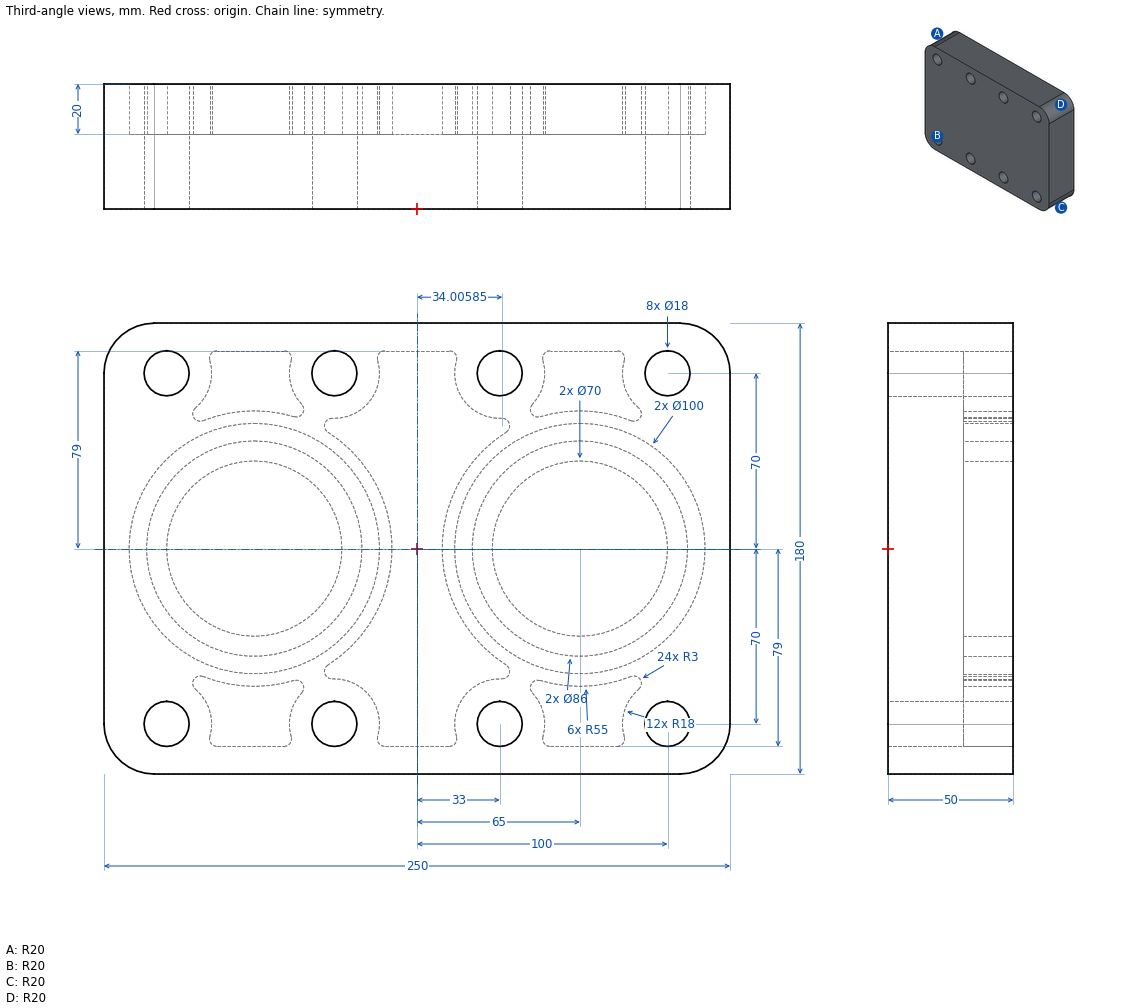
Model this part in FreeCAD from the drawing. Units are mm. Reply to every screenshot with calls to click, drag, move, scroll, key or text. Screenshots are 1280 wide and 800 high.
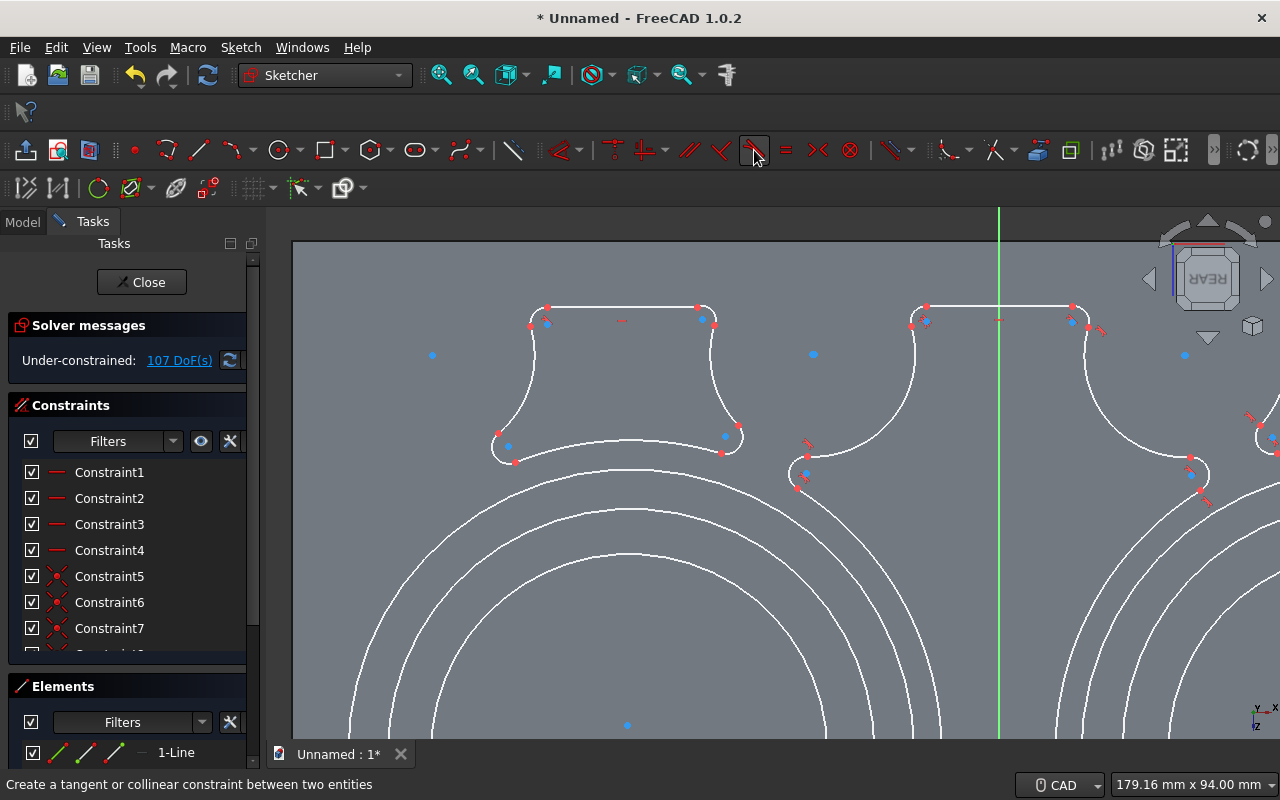
click(652, 307)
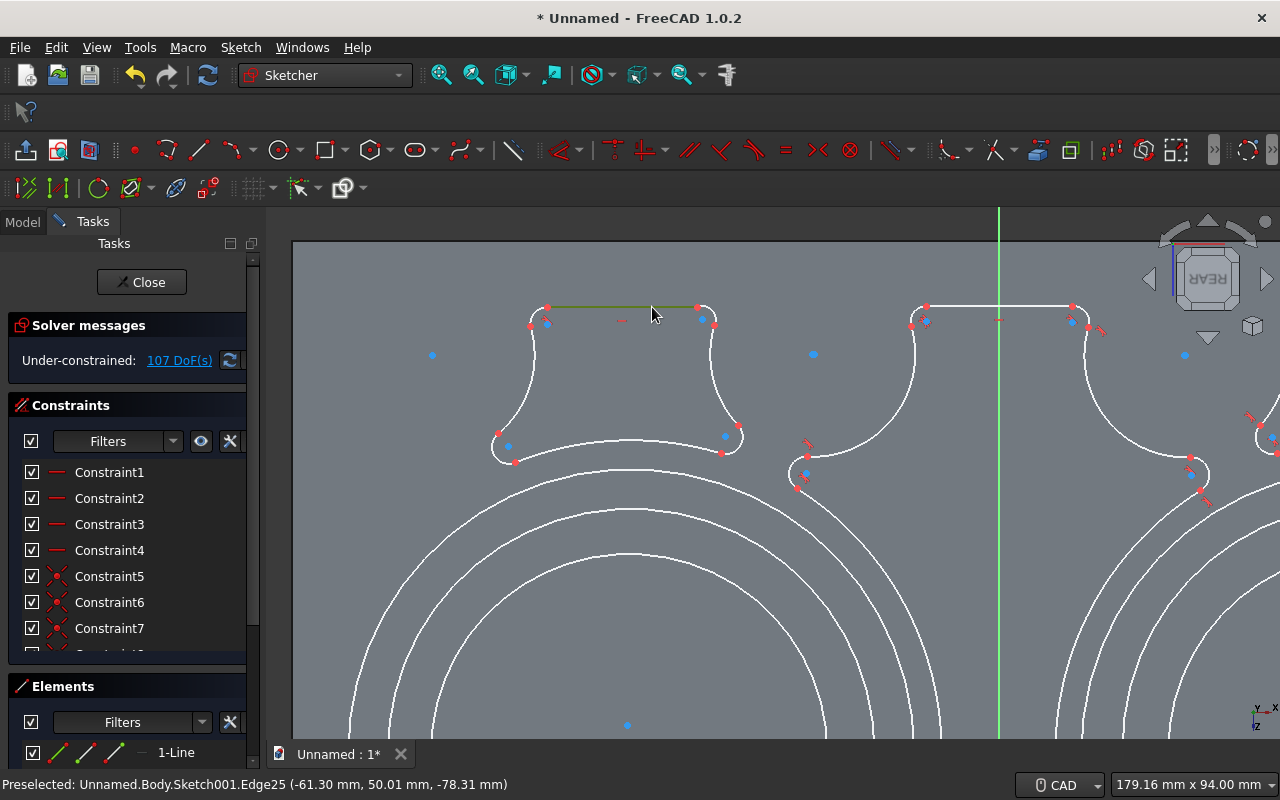
scroll(715, 316, up, 2)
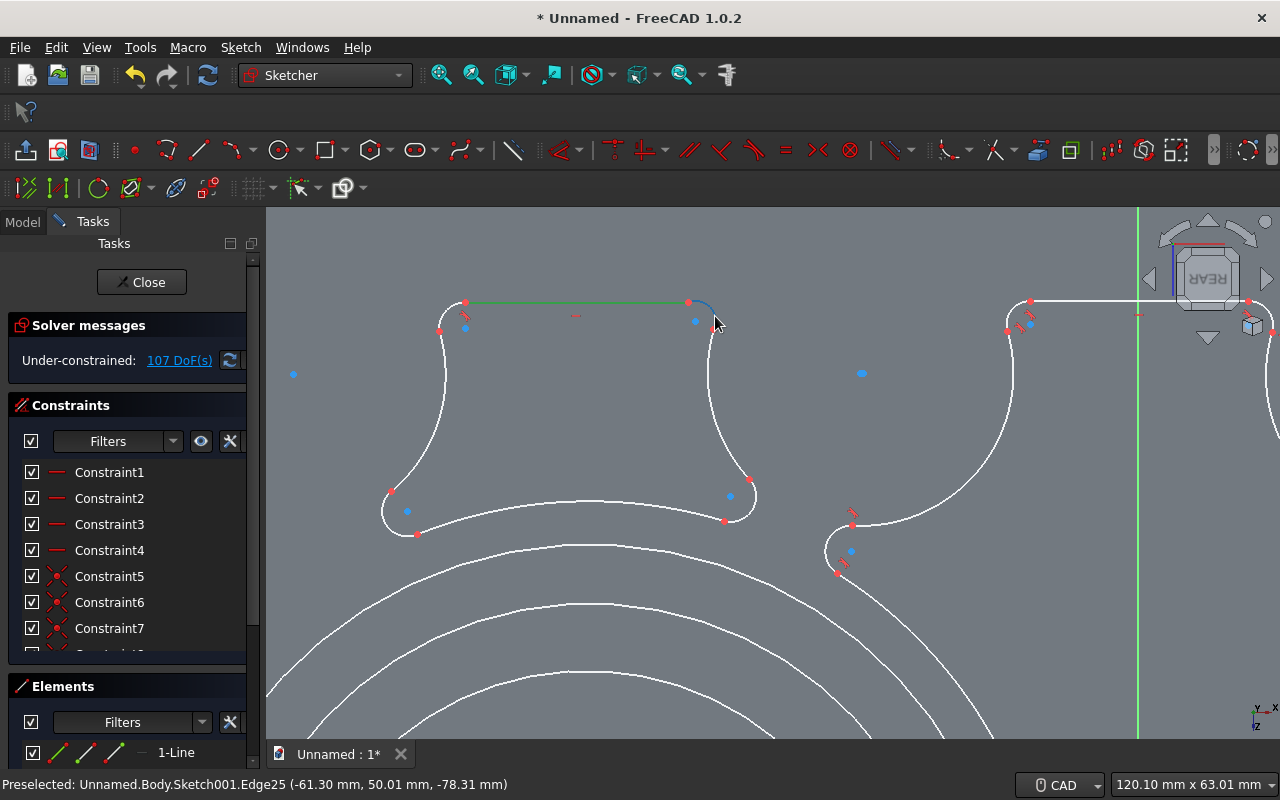
click(715, 316)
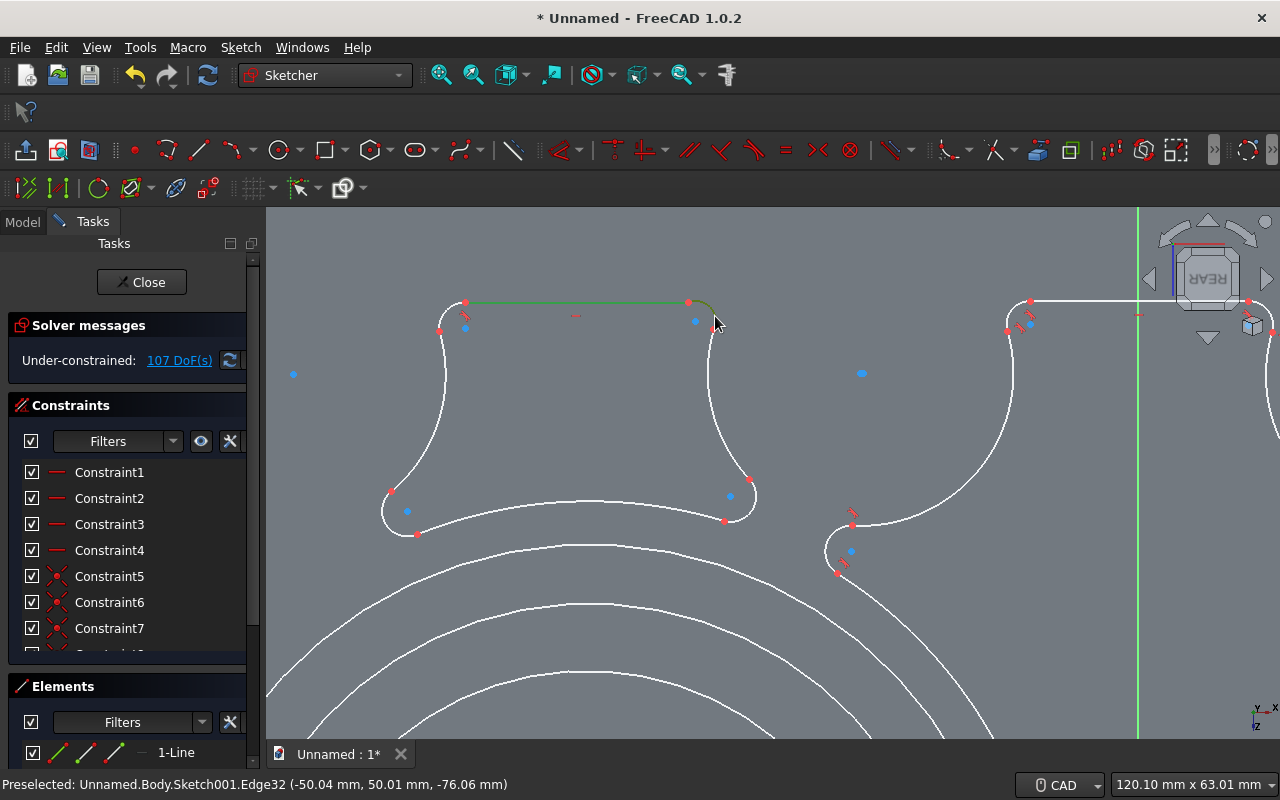
click(754, 150)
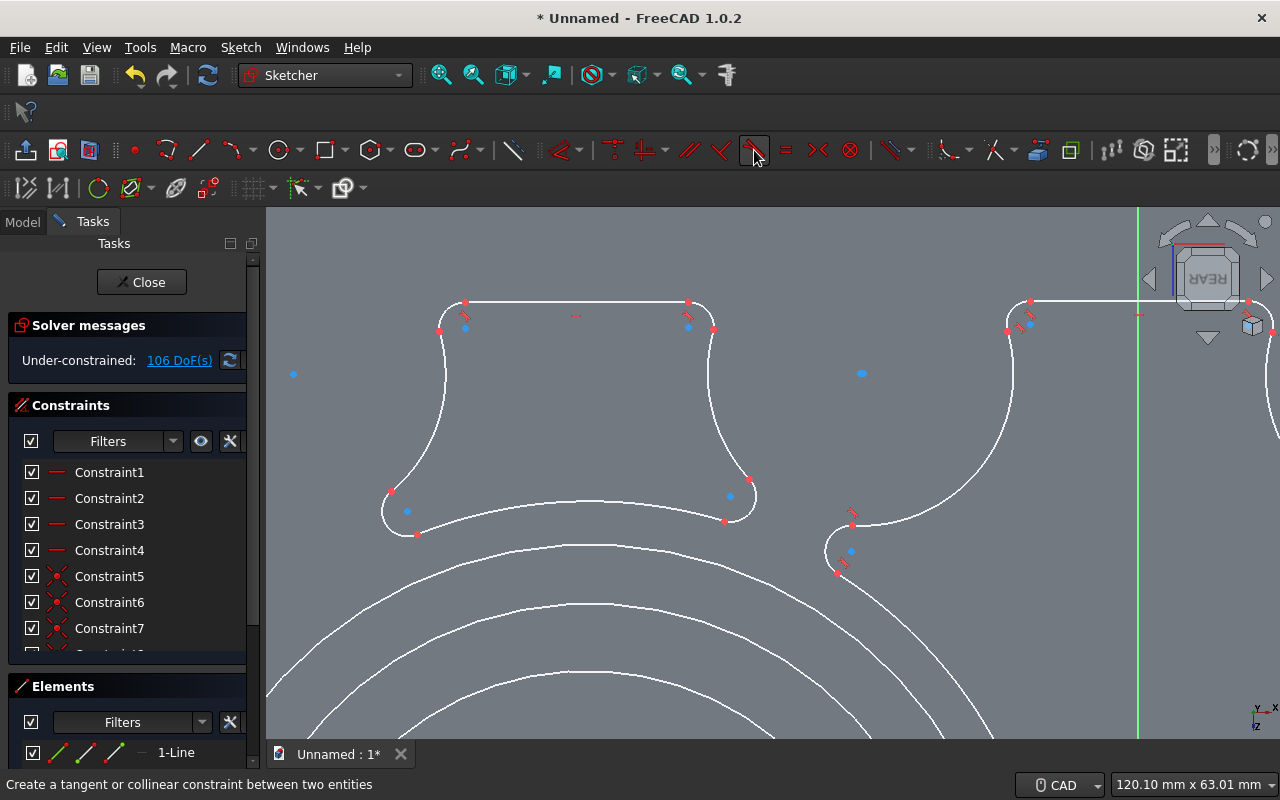
click(452, 306)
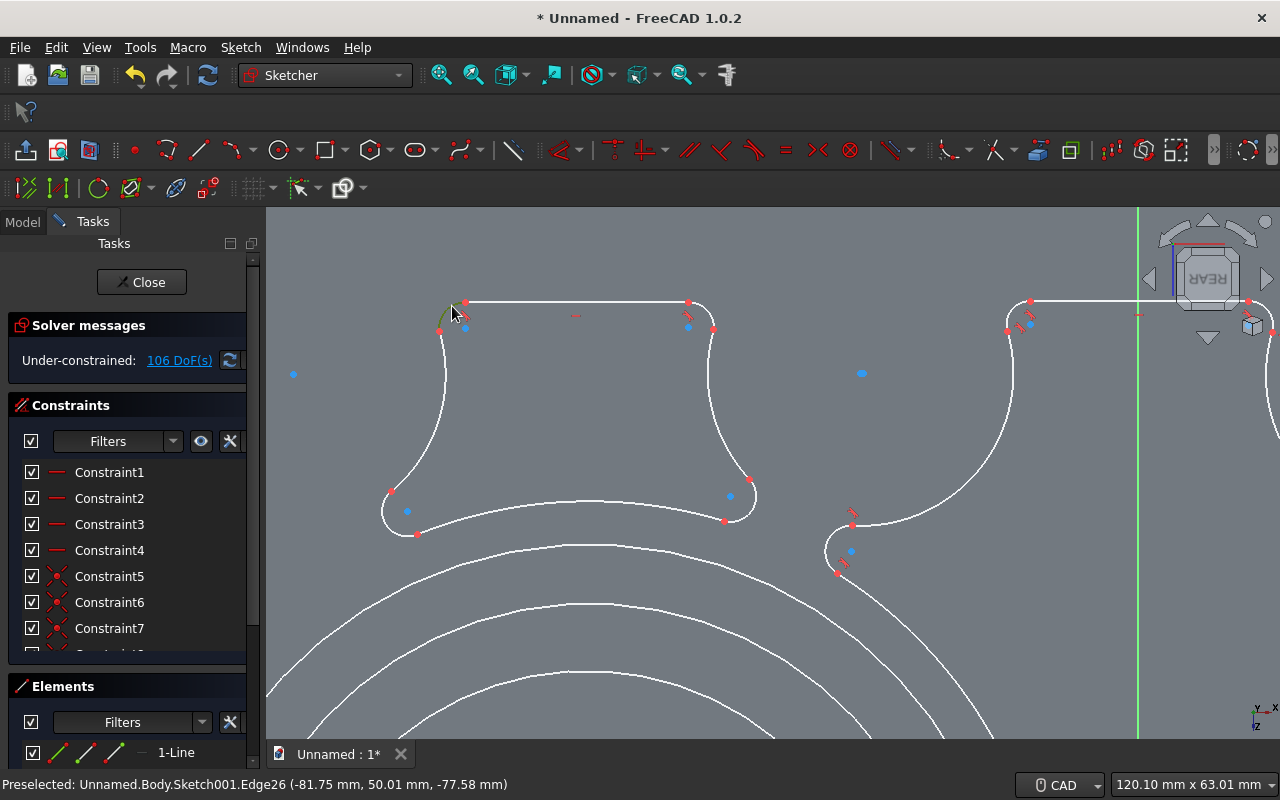
scroll(562, 312, down, 7)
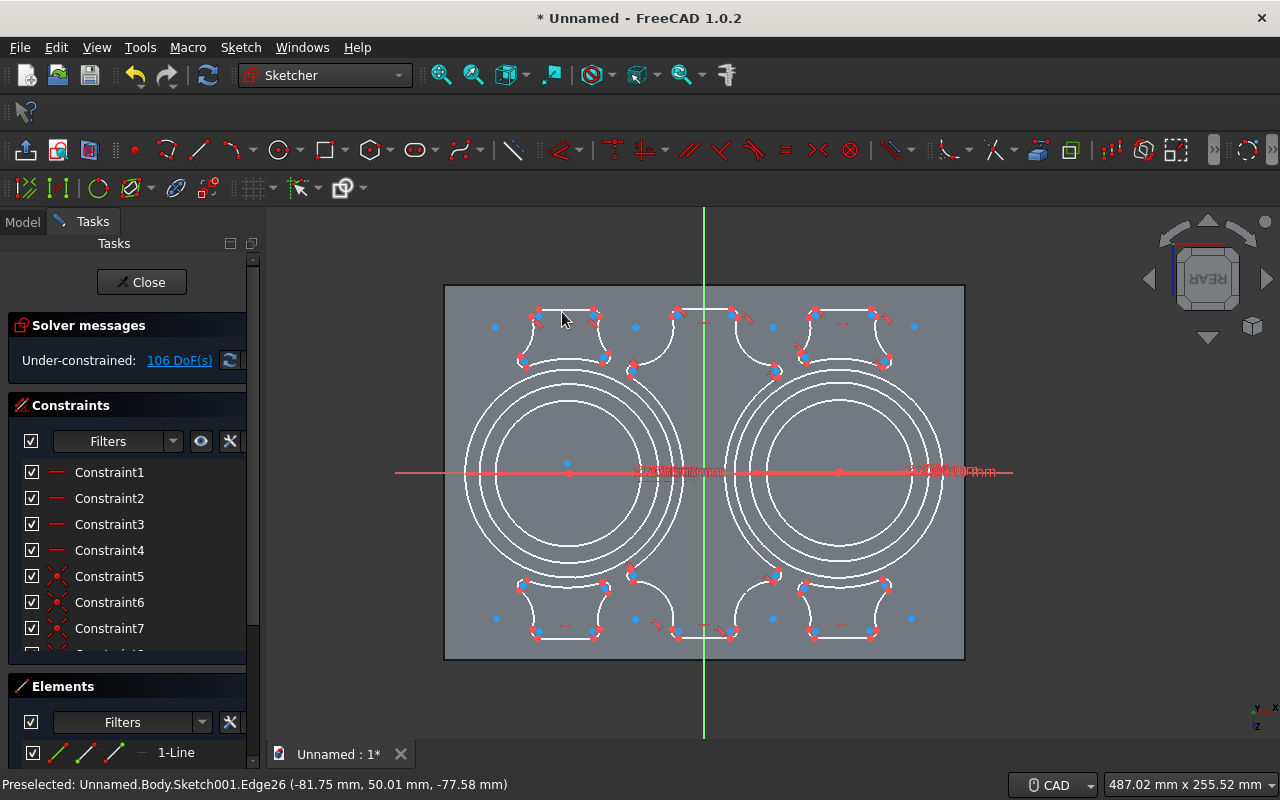
click(529, 346)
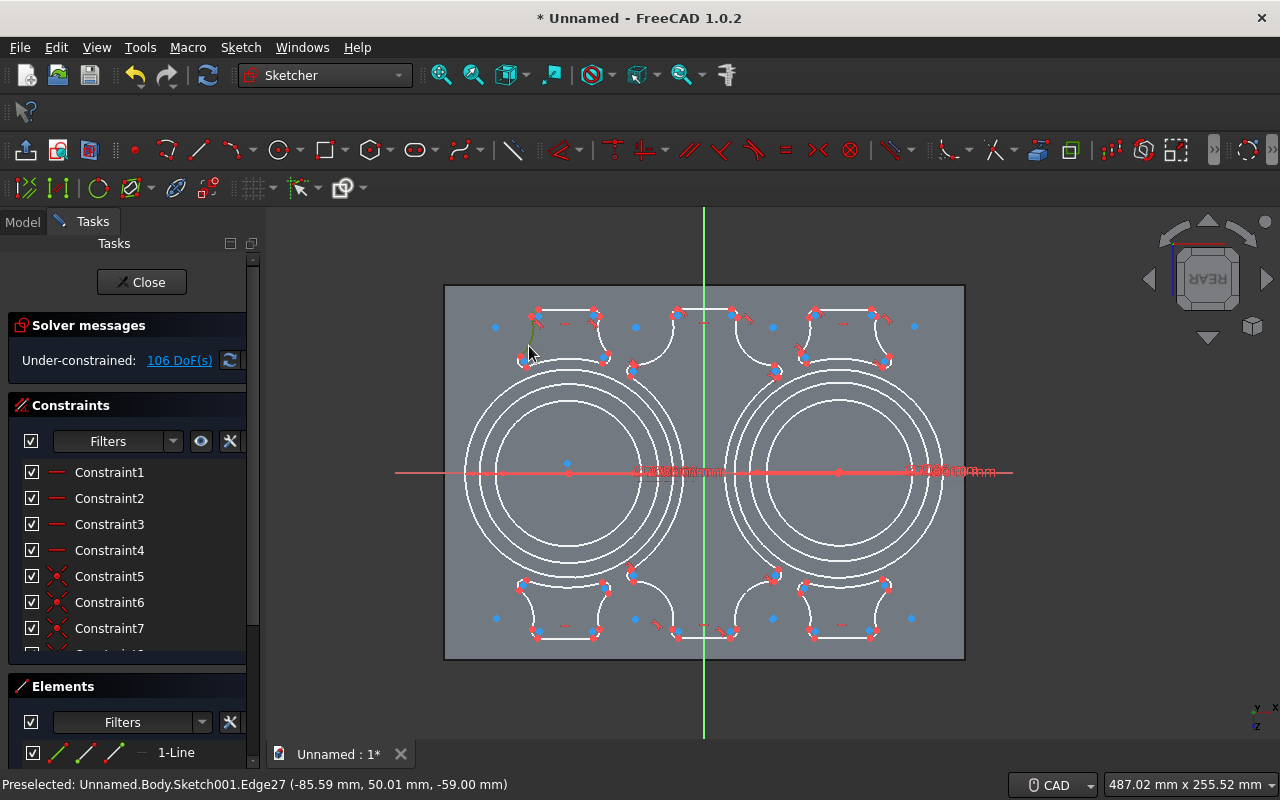
click(754, 150)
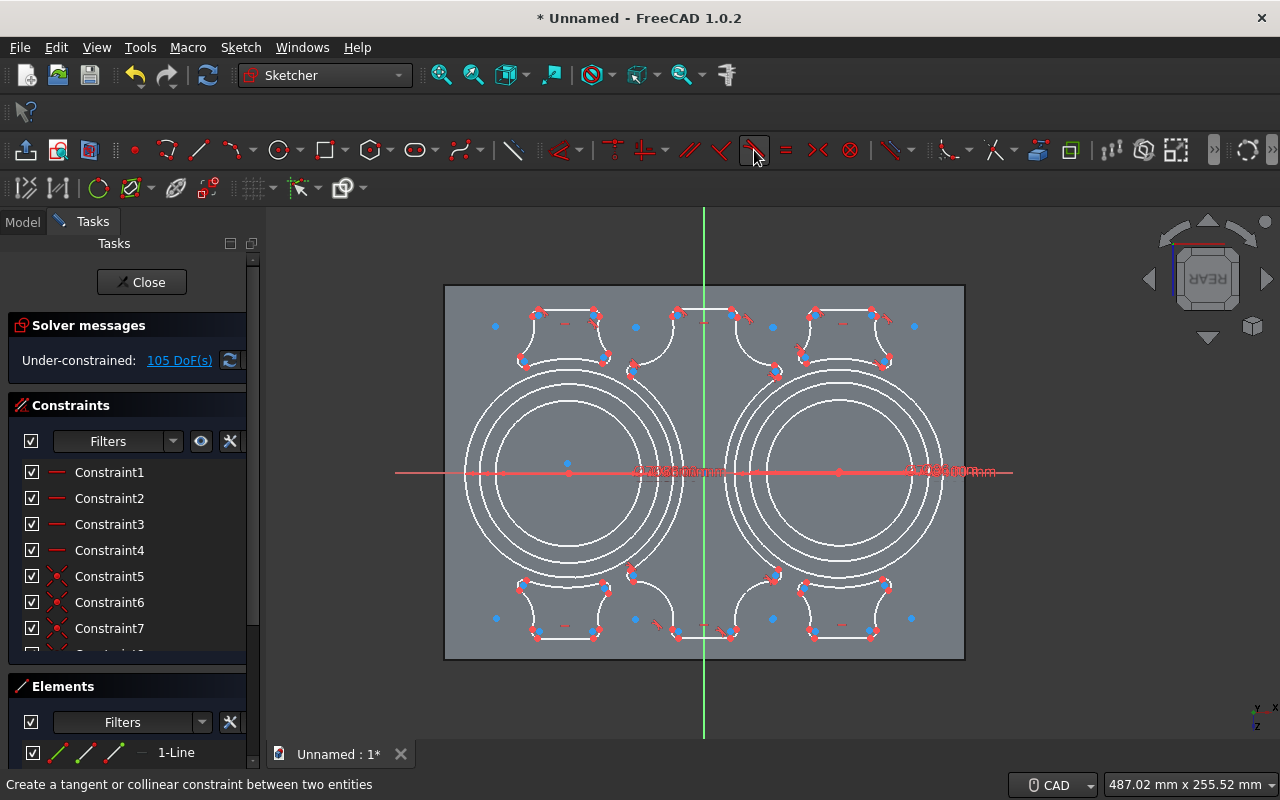
click(529, 346)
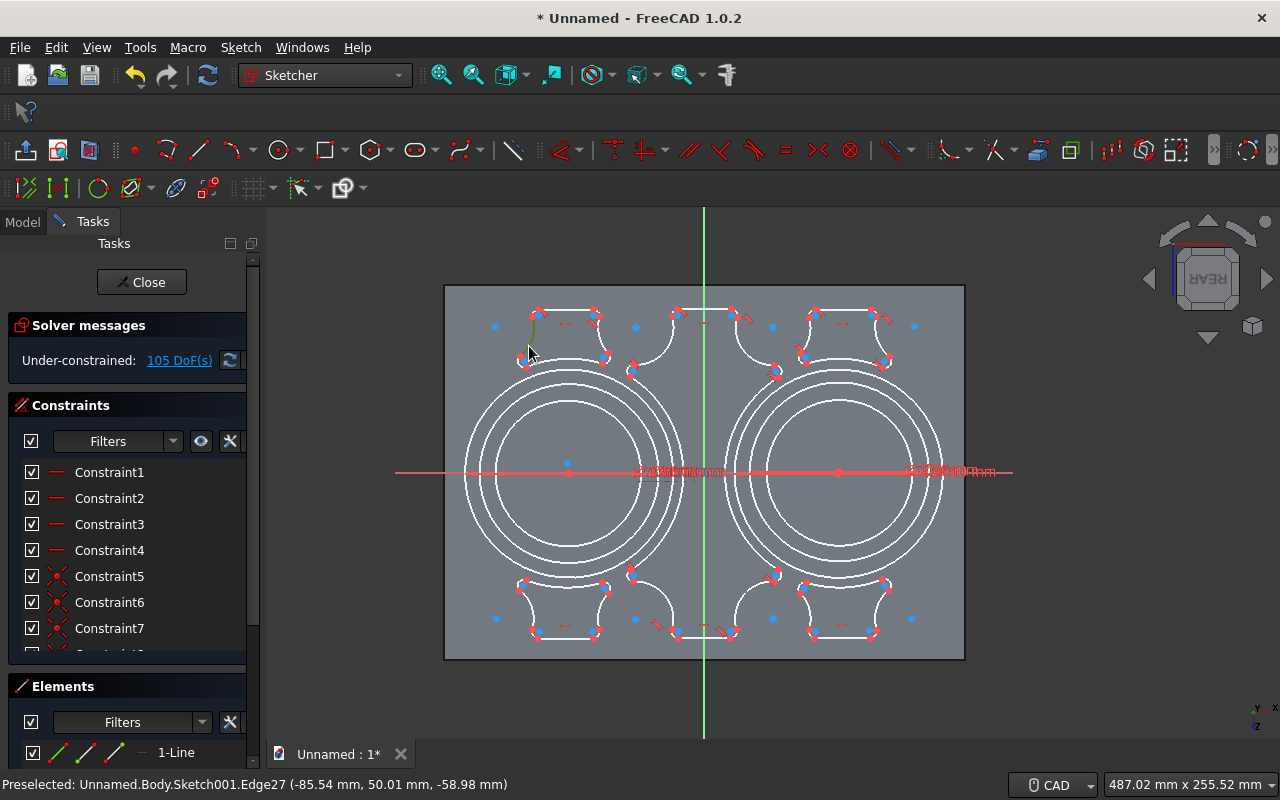
scroll(519, 364, up, 4)